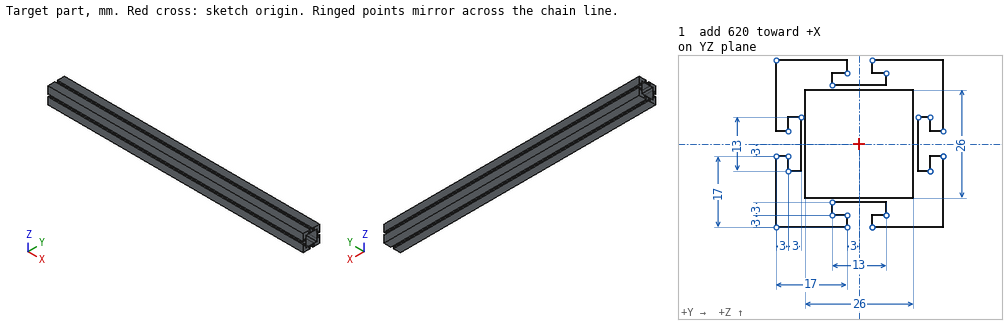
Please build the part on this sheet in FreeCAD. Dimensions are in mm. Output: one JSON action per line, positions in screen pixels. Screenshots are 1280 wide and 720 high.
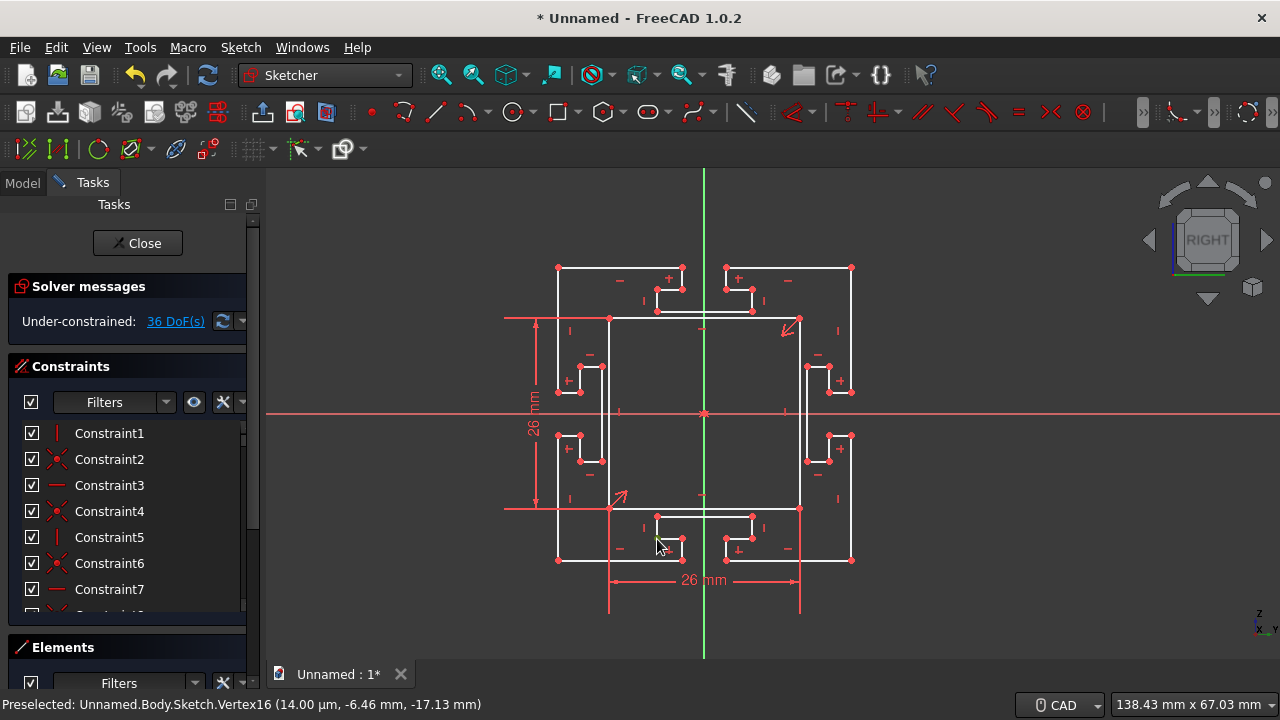
{"action": "left_click", "coordinate": [752, 539]}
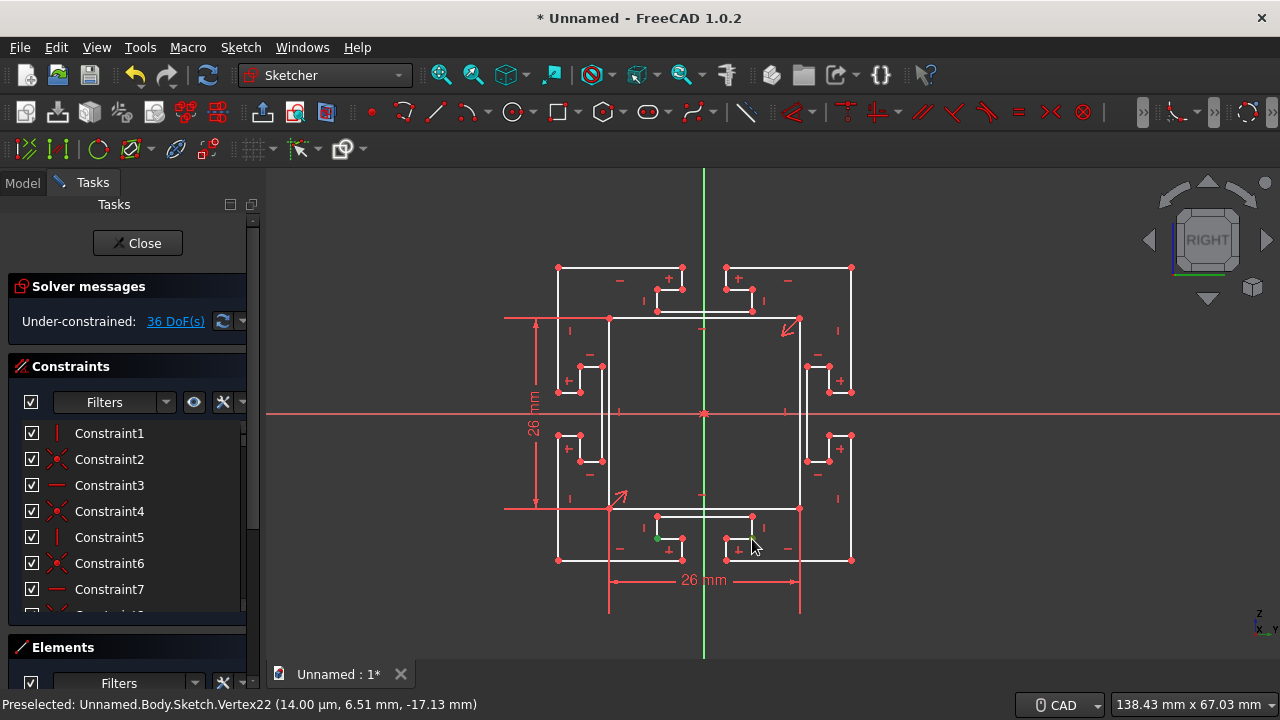
{"action": "left_click", "coordinate": [704, 600]}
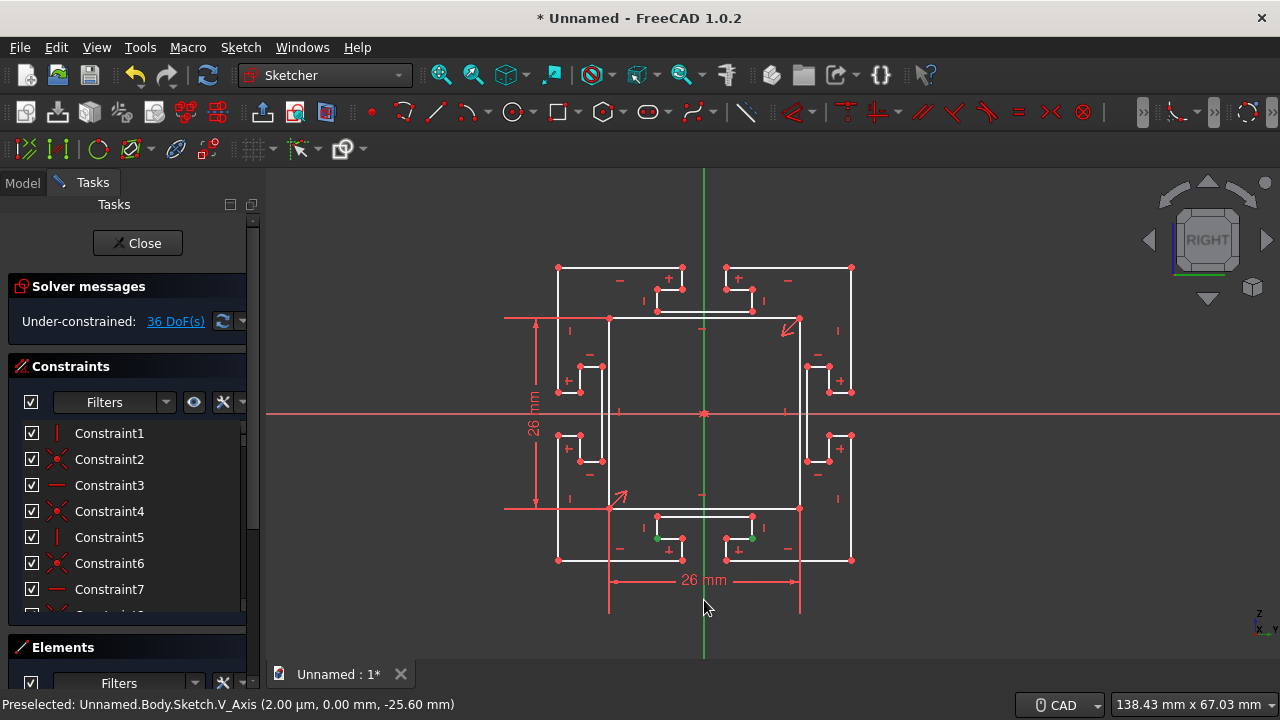
{"action": "key", "text": "s"}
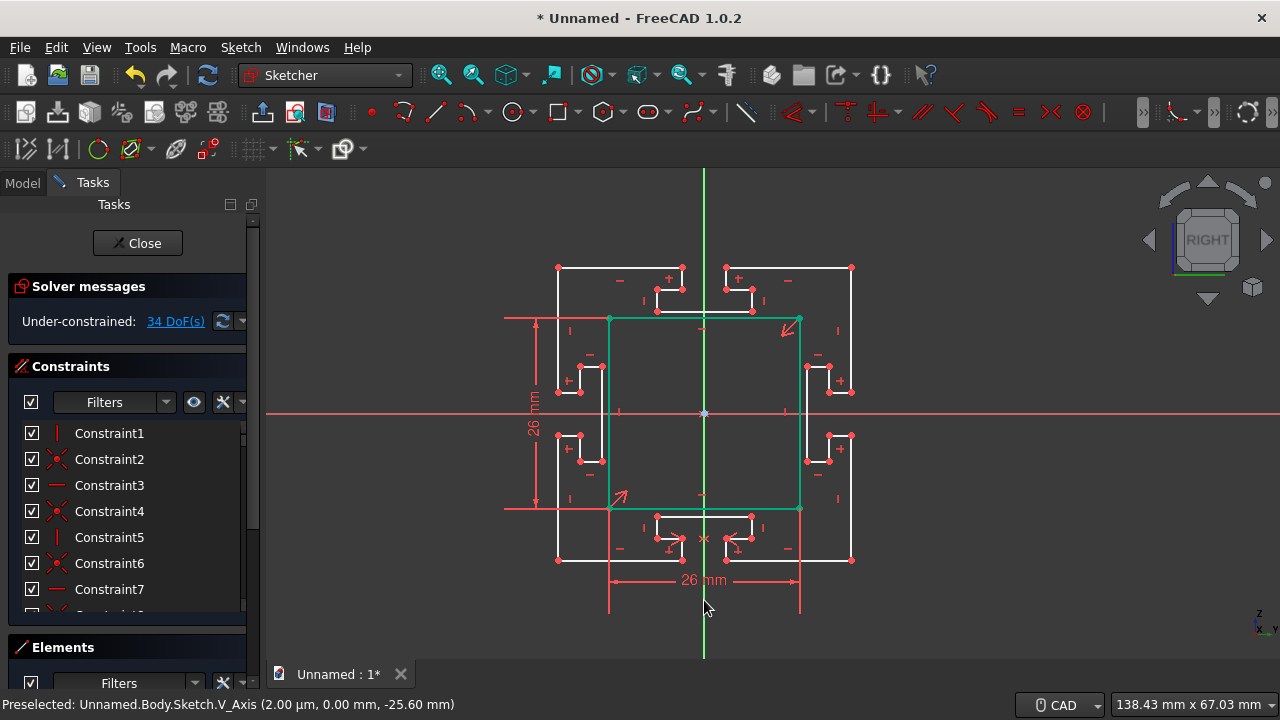
{"action": "left_click", "coordinate": [682, 561]}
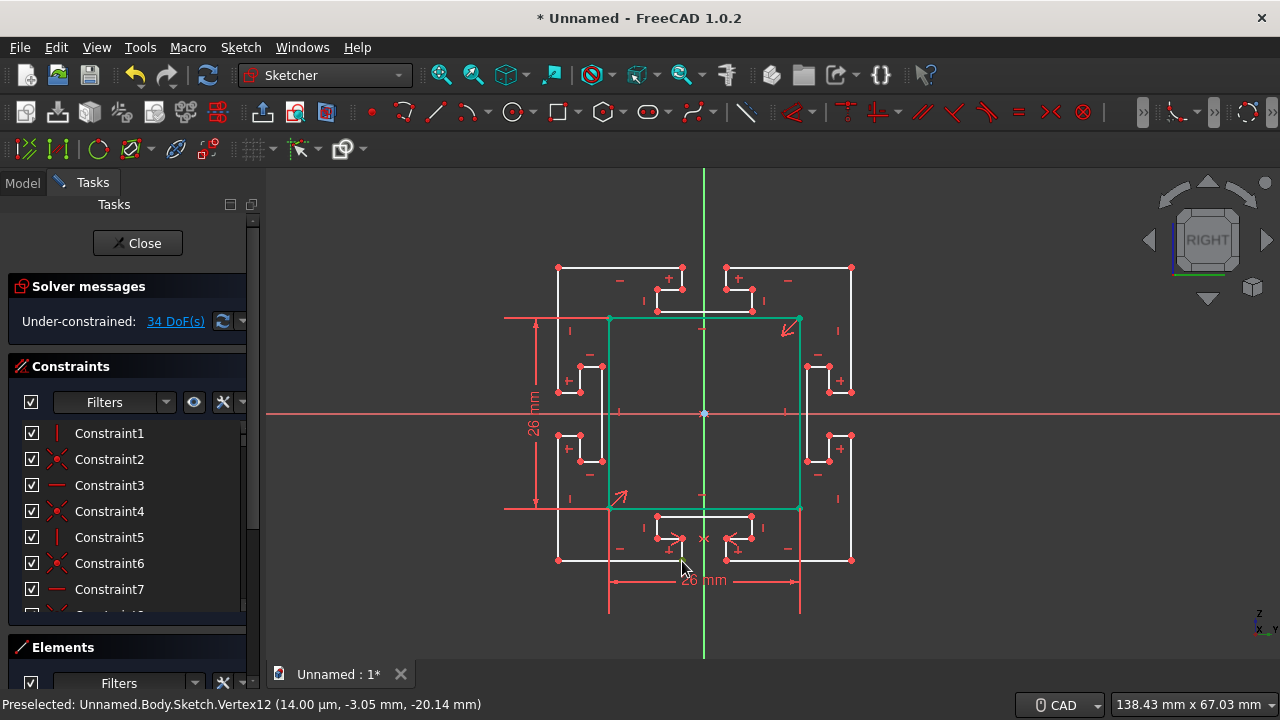
{"action": "left_click", "coordinate": [726, 561]}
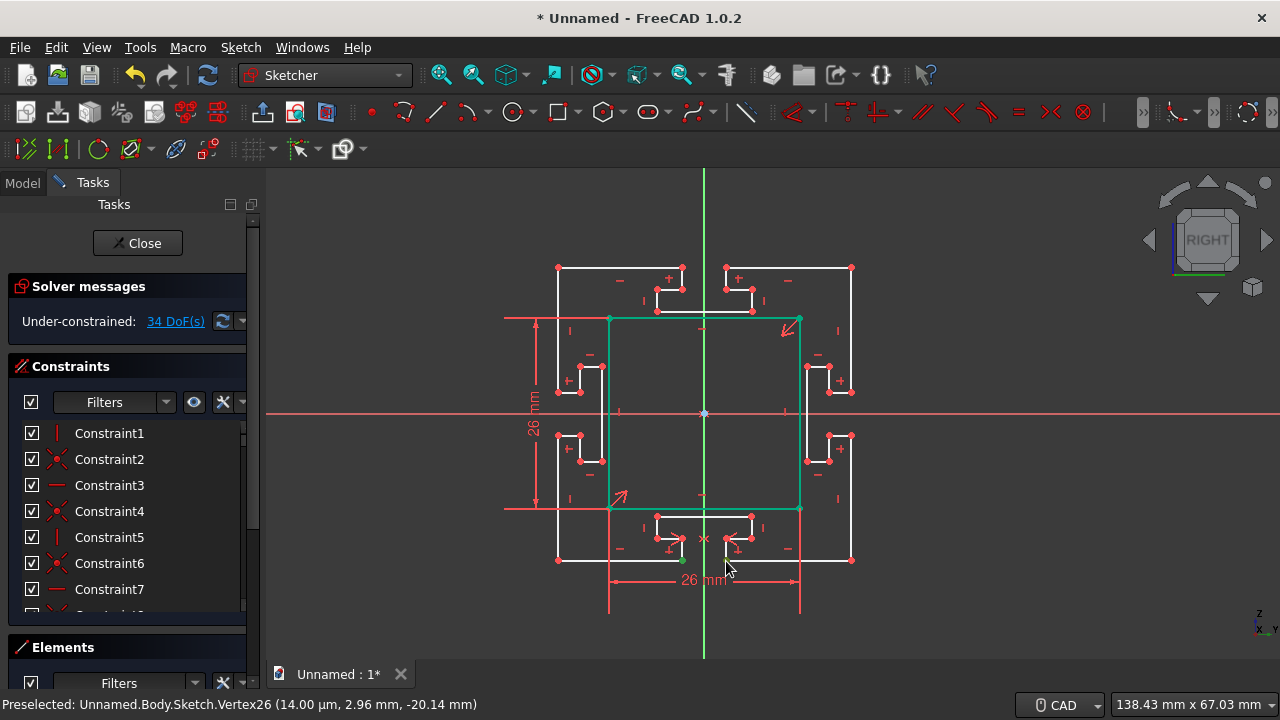
{"action": "left_click", "coordinate": [704, 600]}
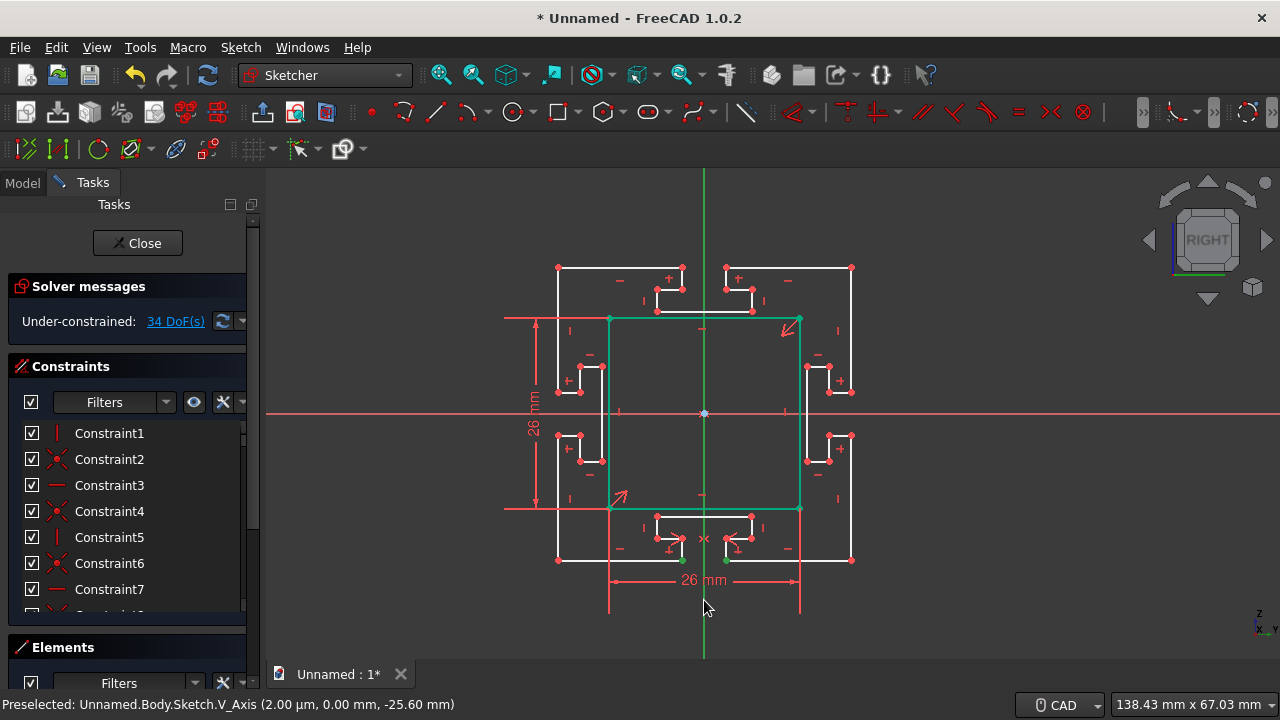
{"action": "key", "text": "s"}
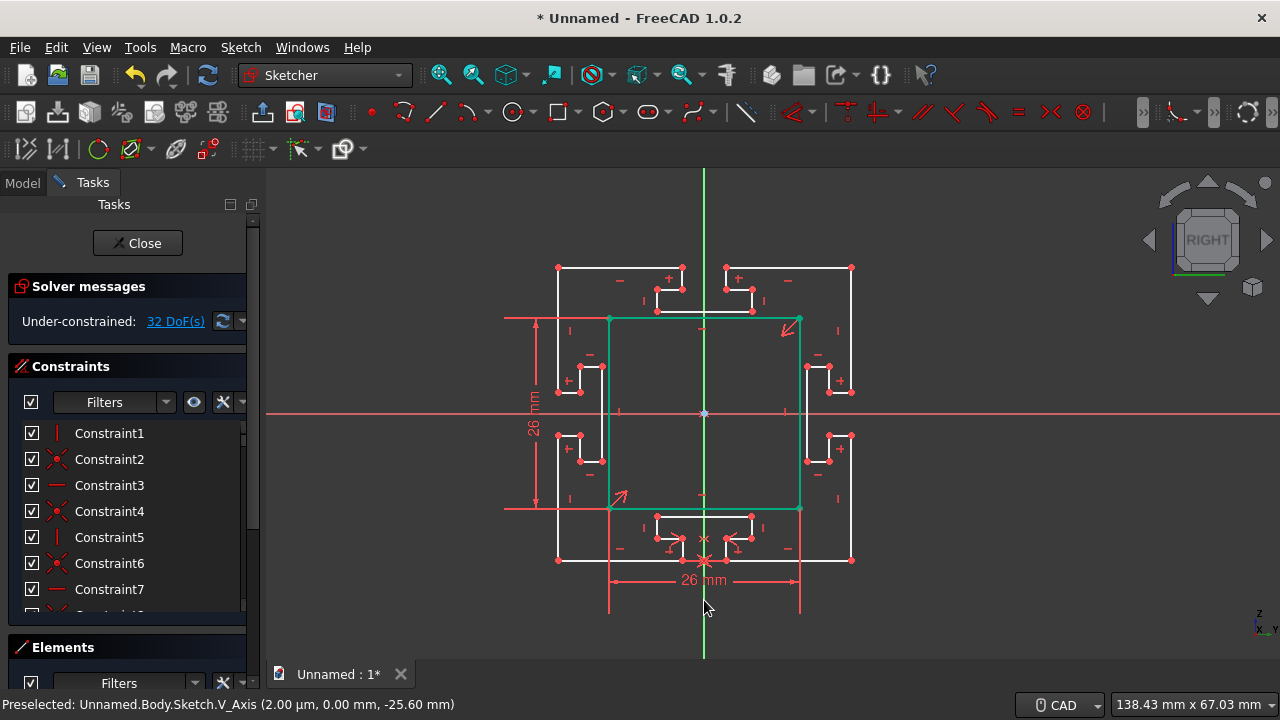
{"action": "left_click", "coordinate": [558, 436]}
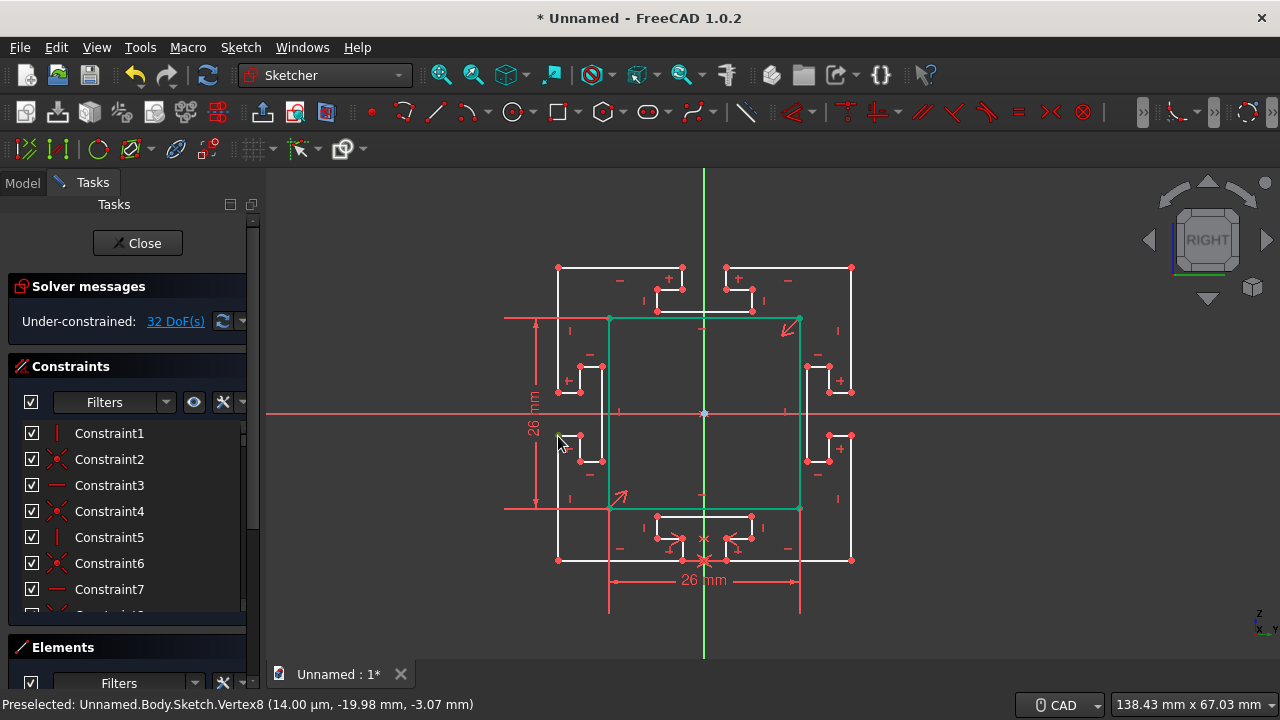
{"action": "left_click", "coordinate": [851, 436]}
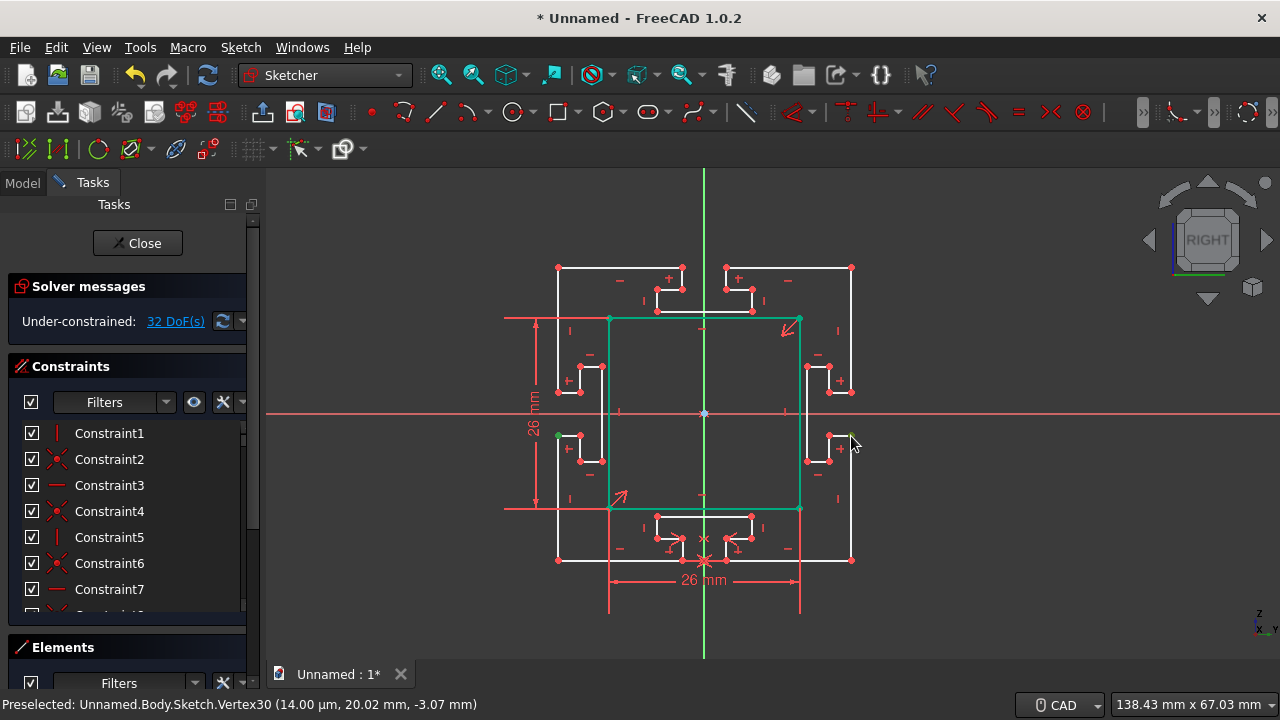
{"action": "left_click", "coordinate": [704, 600]}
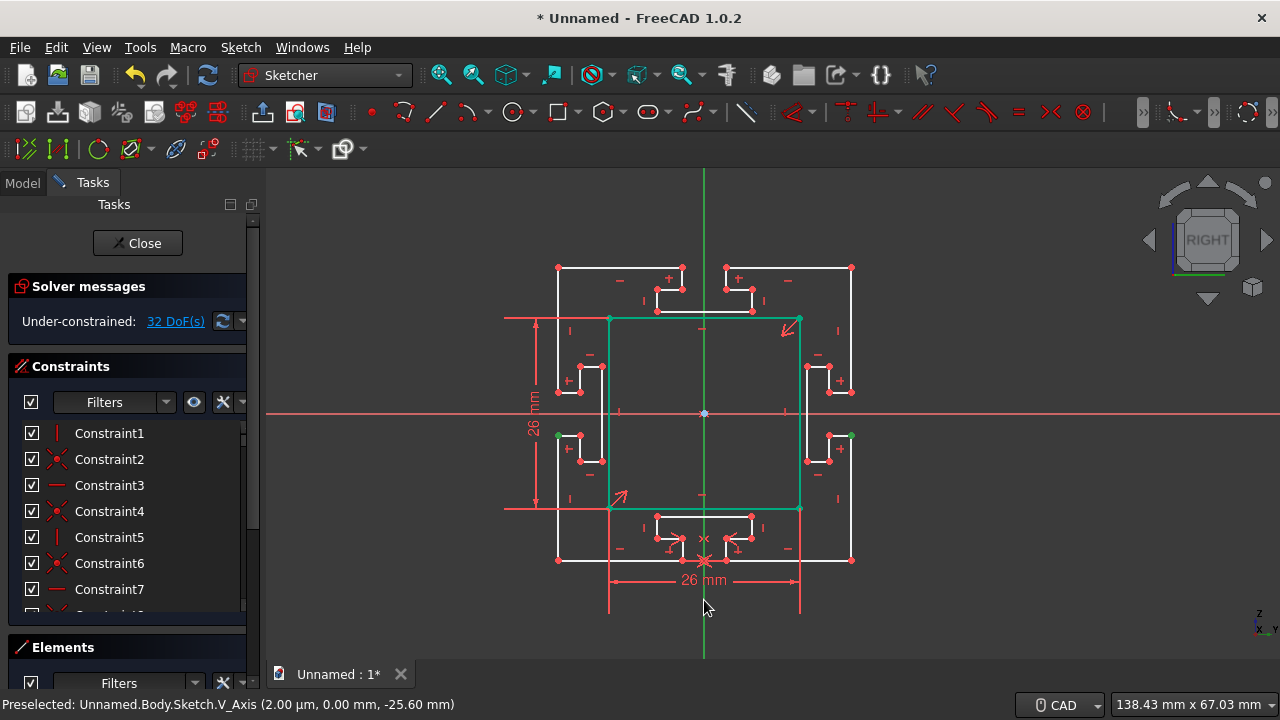
{"action": "key", "text": "s"}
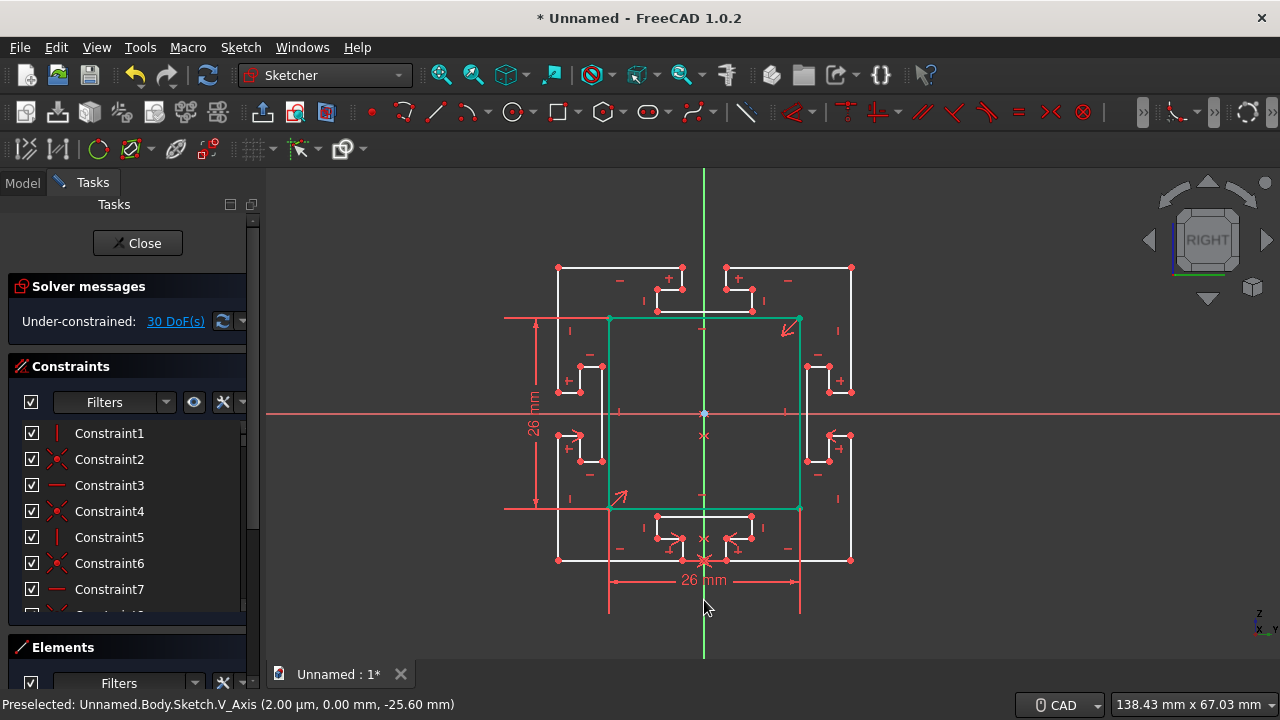
{"action": "left_click", "coordinate": [580, 462]}